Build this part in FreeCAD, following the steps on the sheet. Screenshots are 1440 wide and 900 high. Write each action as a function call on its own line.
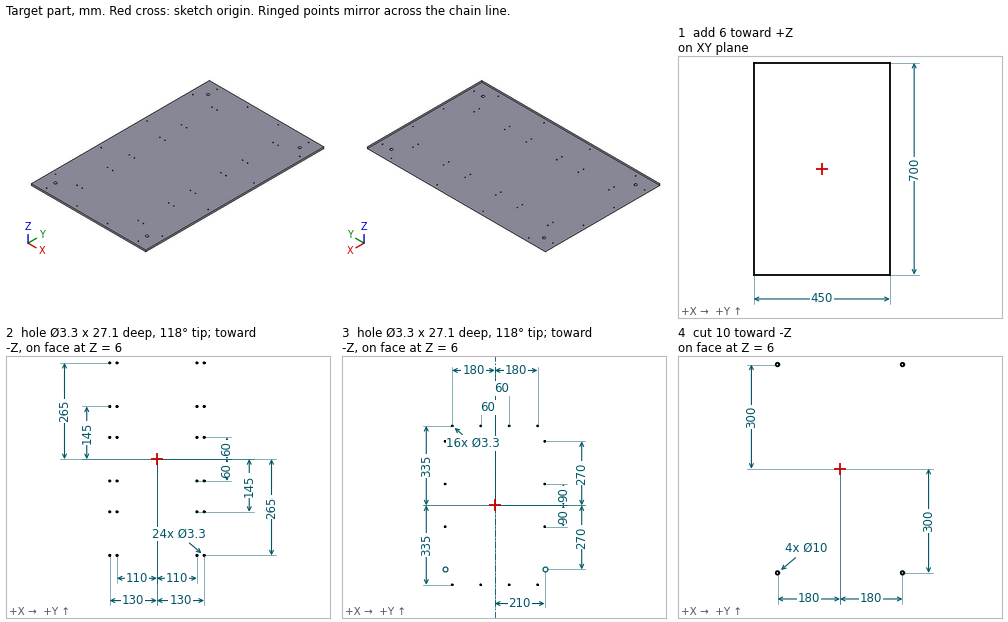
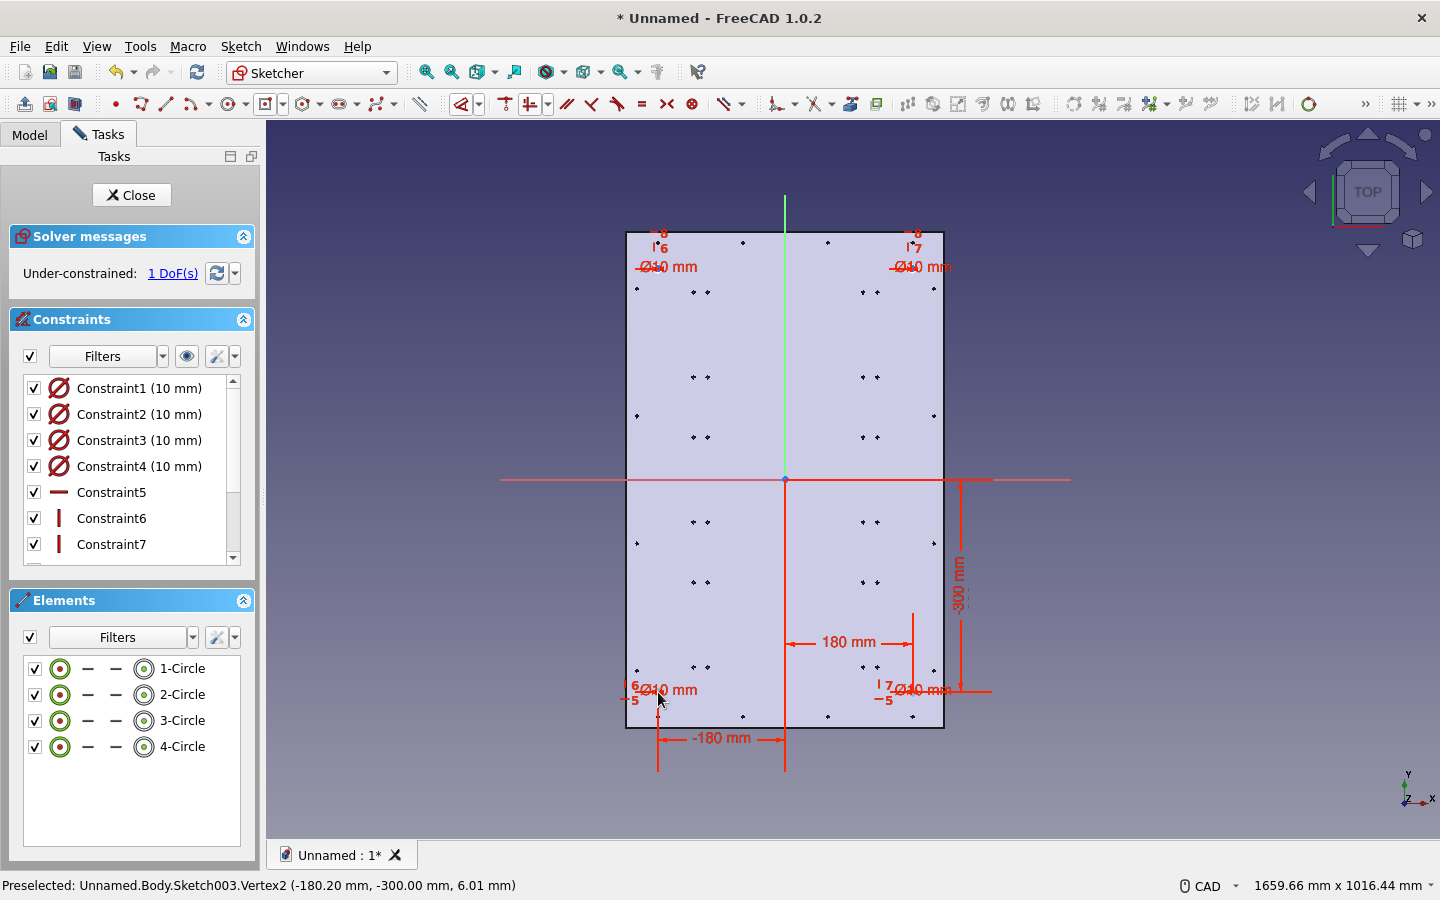
click(658, 269)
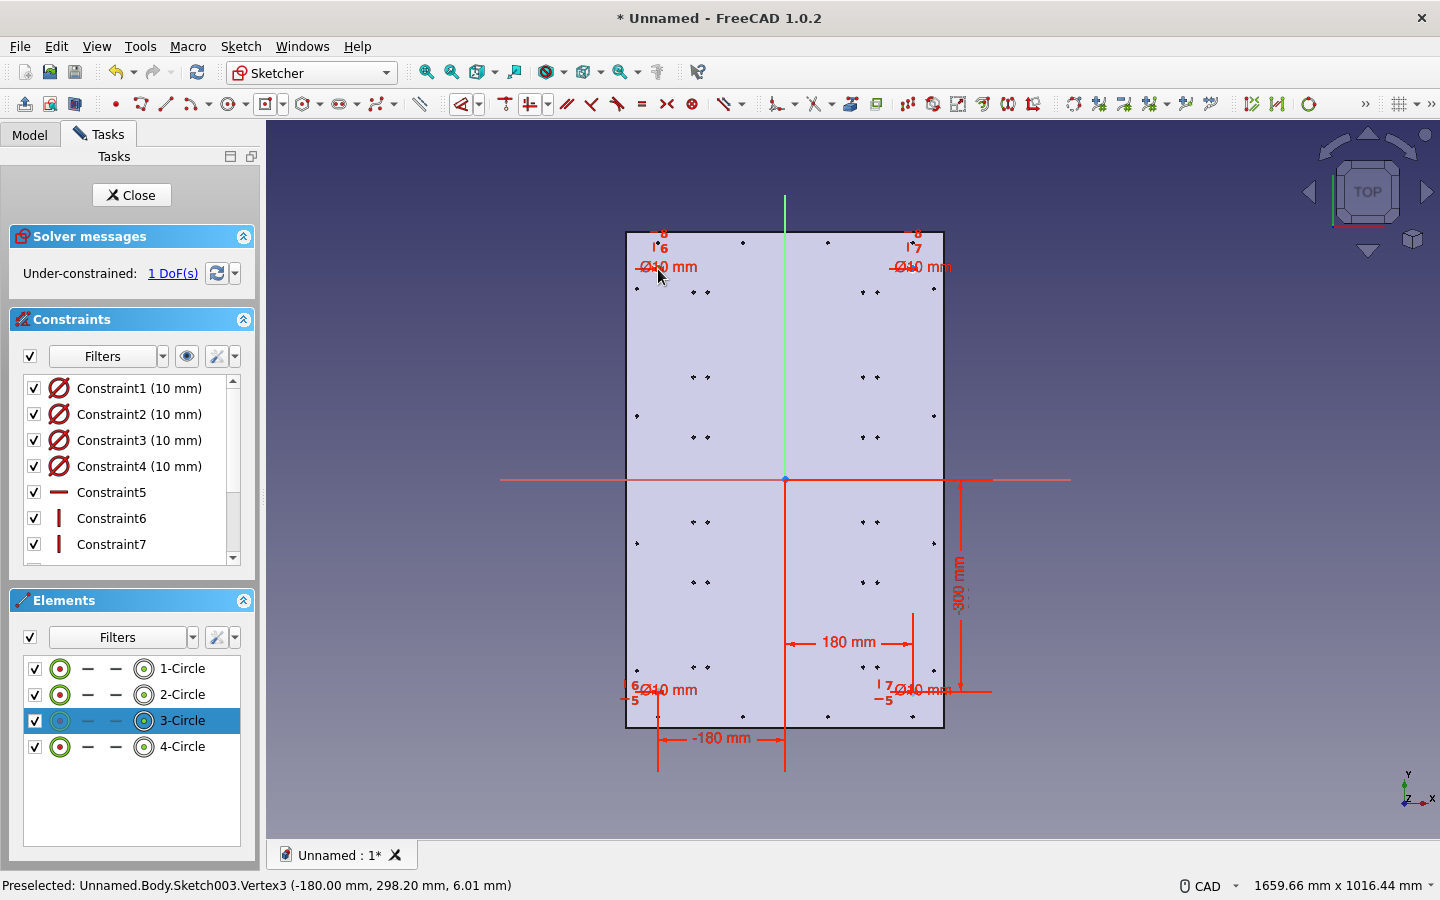
key(i)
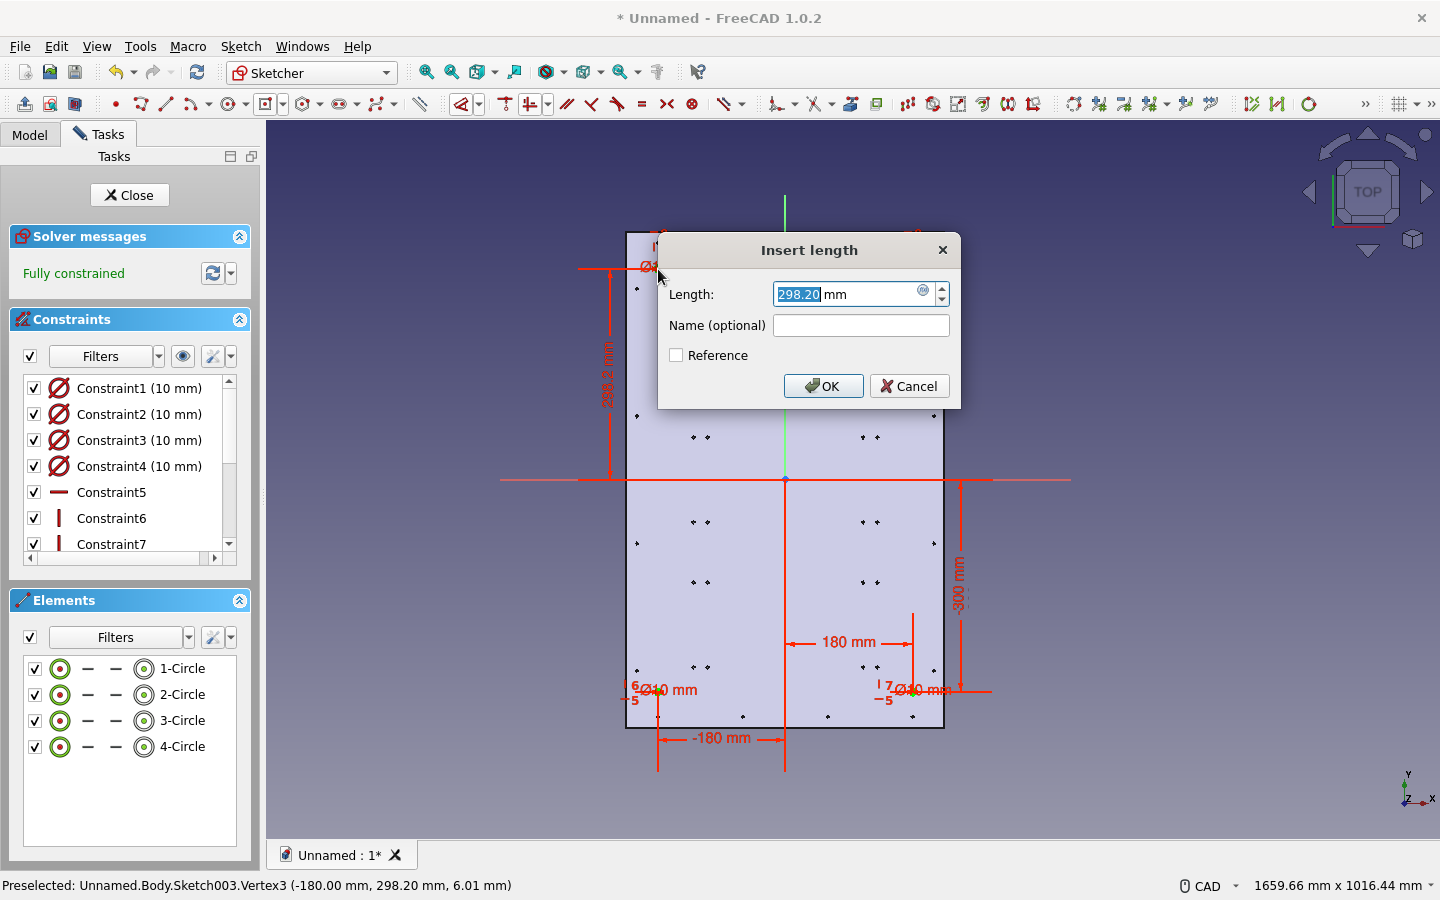
text(300)
key(Return)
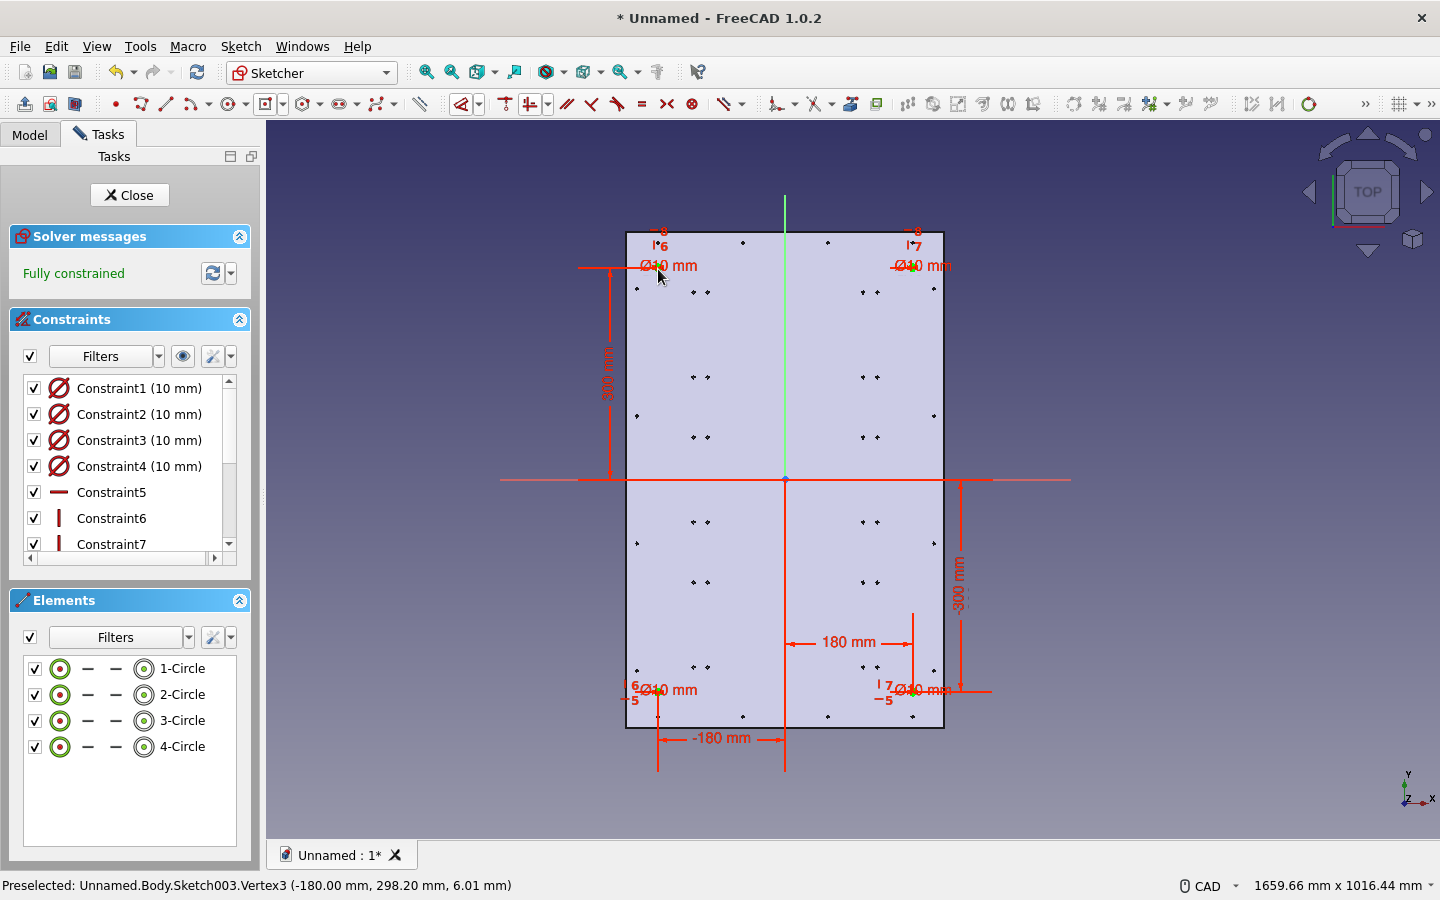
click(130, 195)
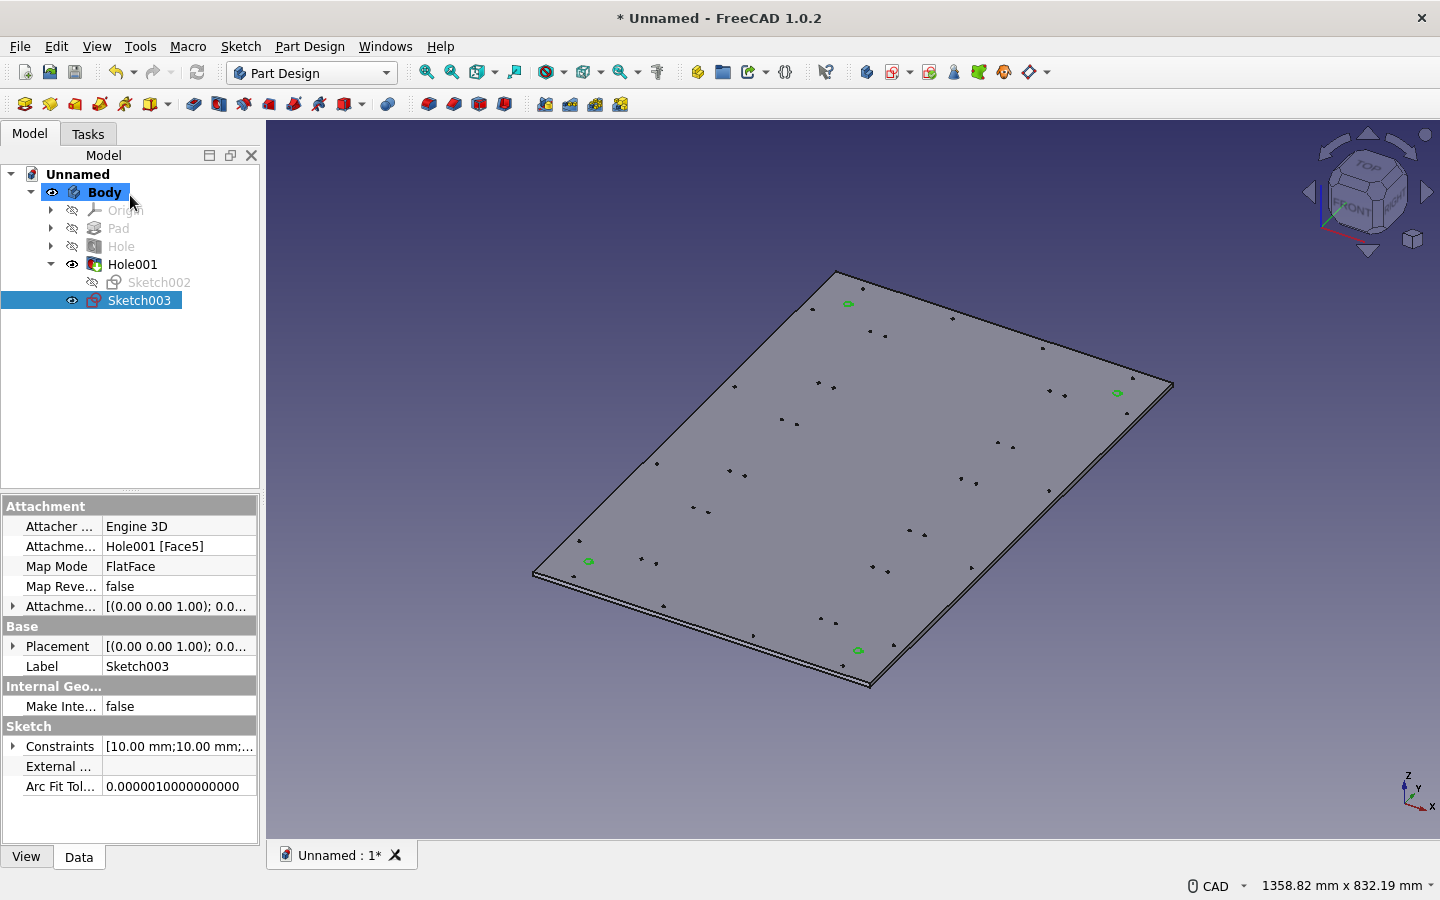
click(194, 104)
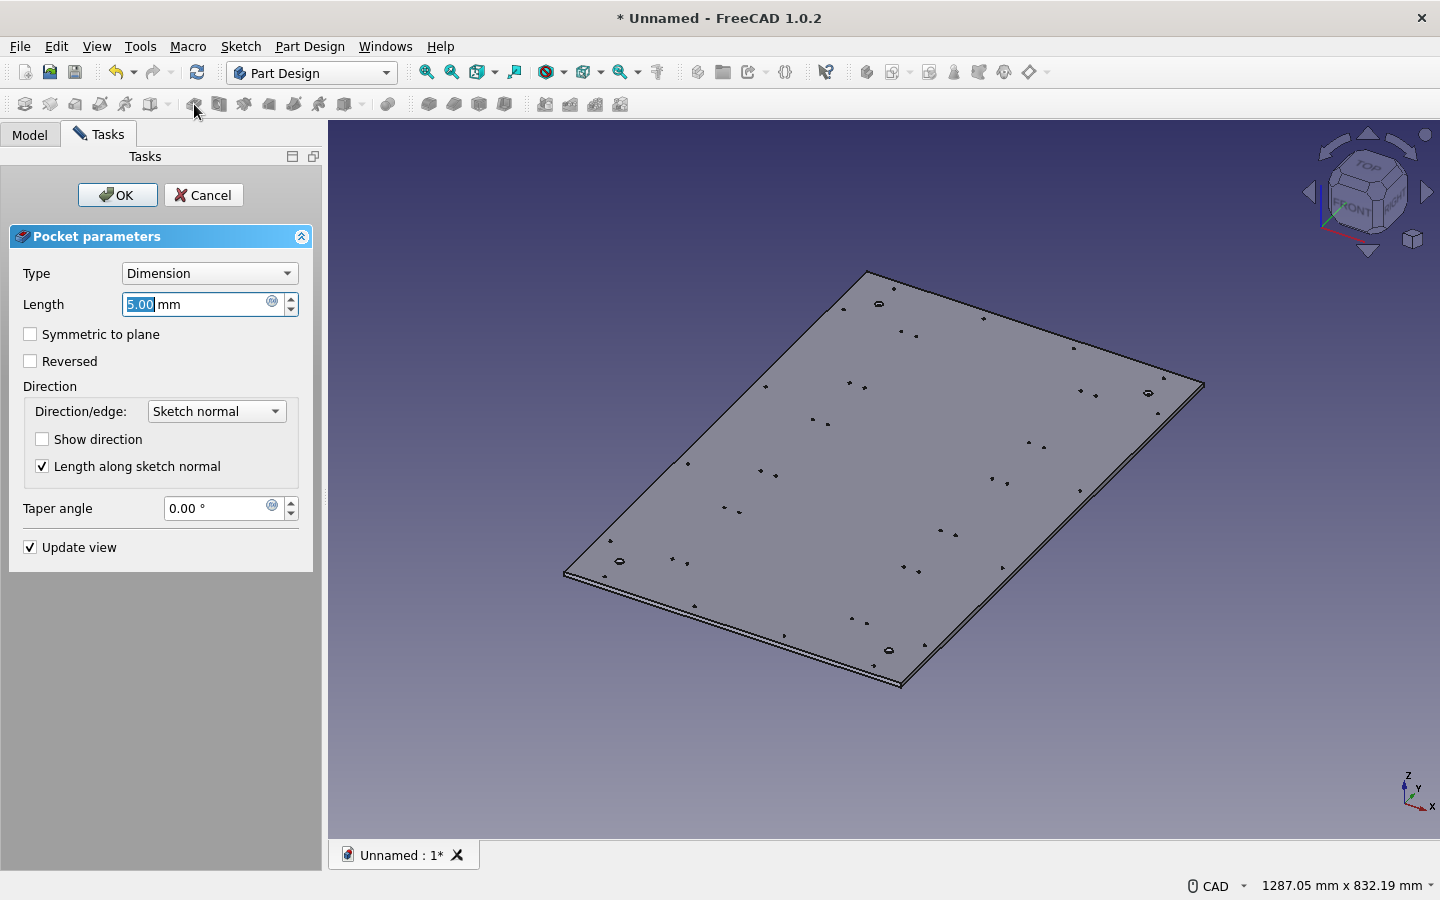
text(10)
key(Tab)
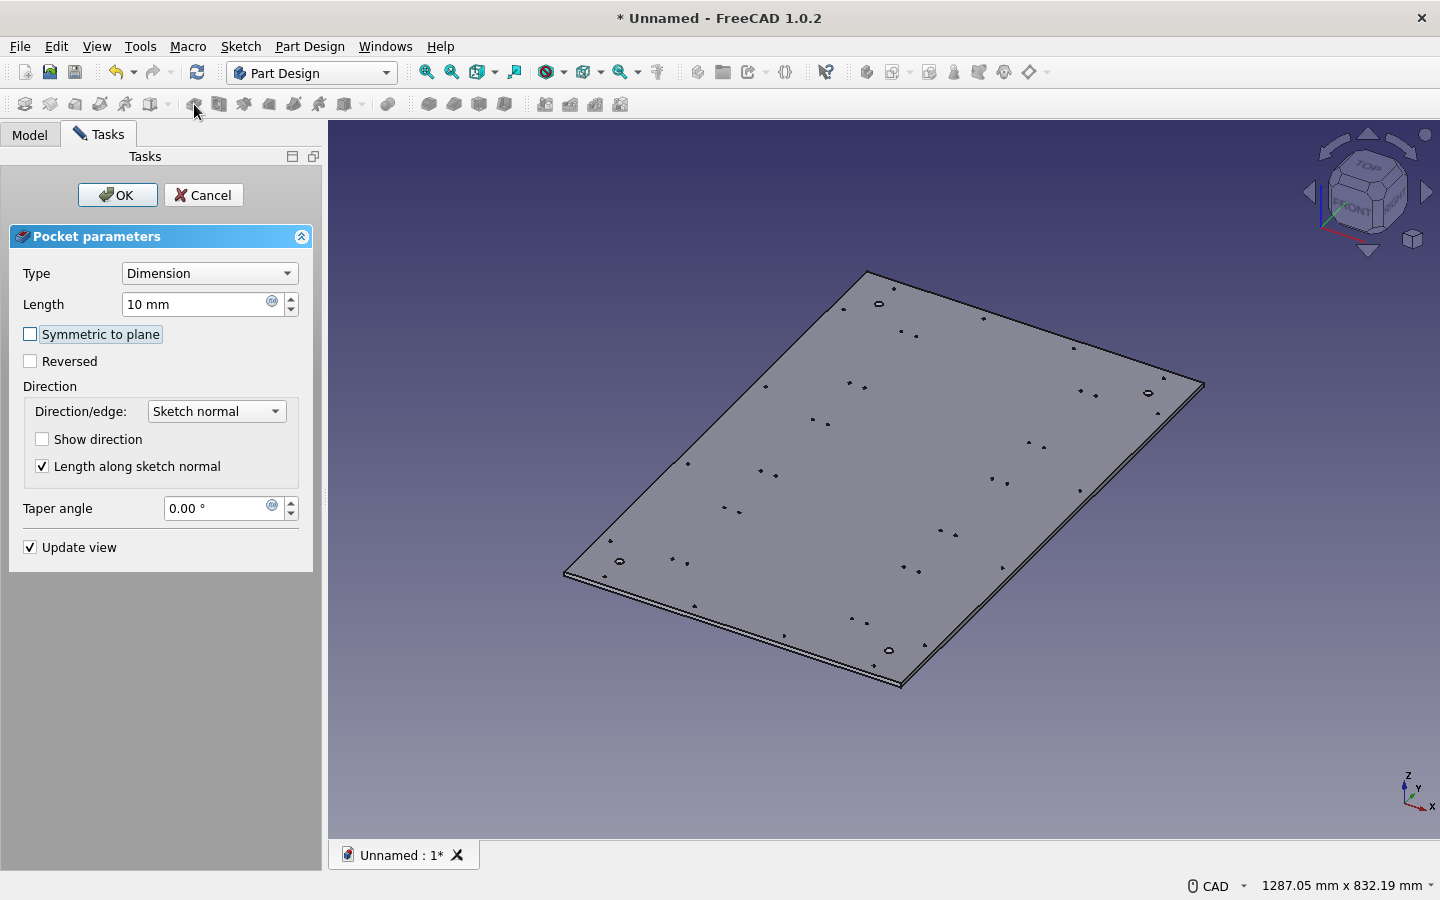
click(118, 195)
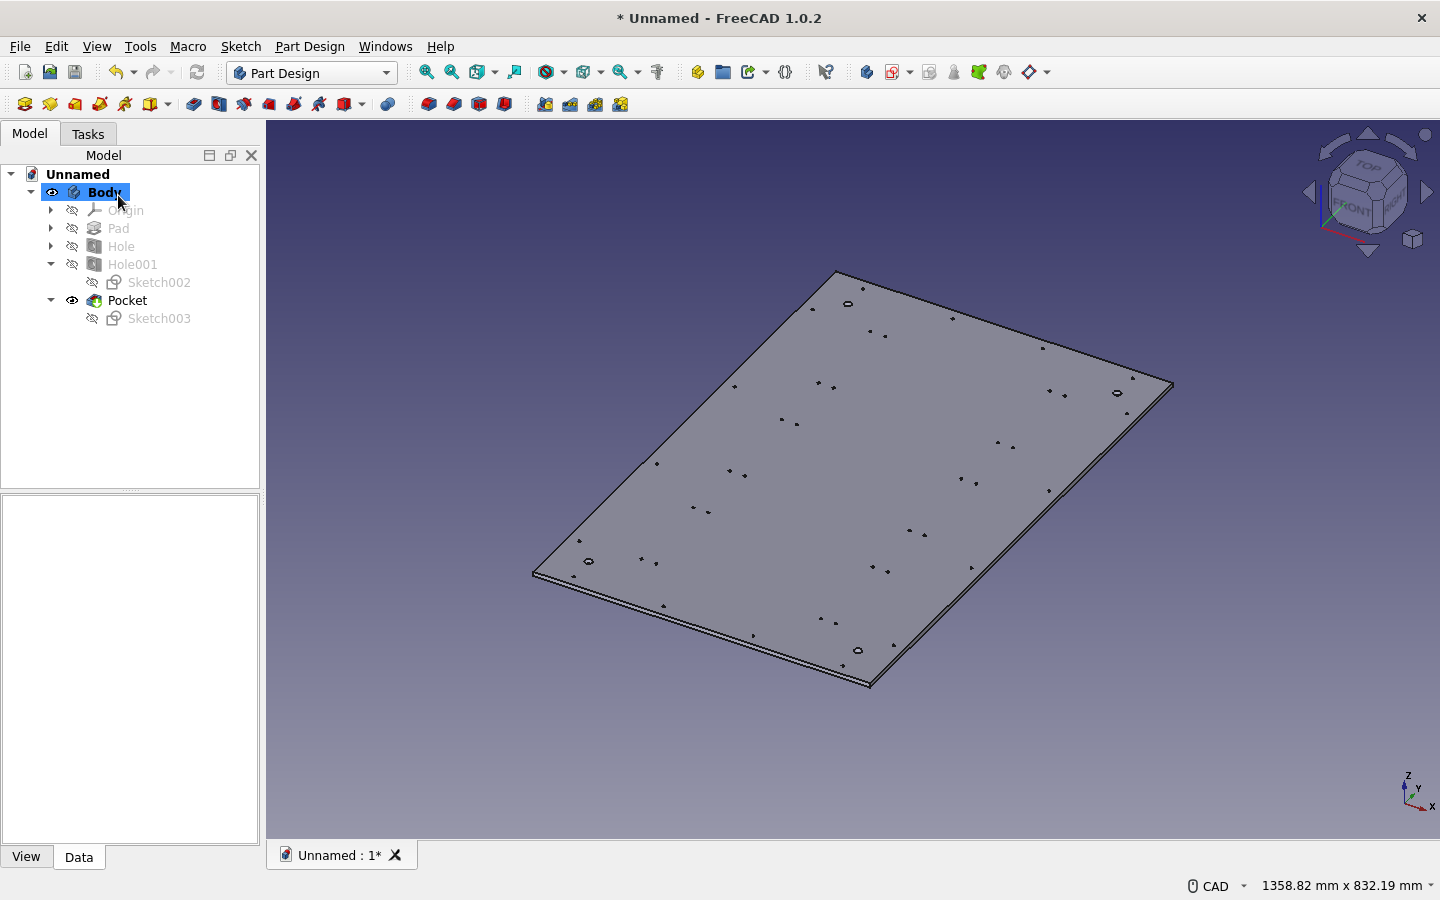
key(0)